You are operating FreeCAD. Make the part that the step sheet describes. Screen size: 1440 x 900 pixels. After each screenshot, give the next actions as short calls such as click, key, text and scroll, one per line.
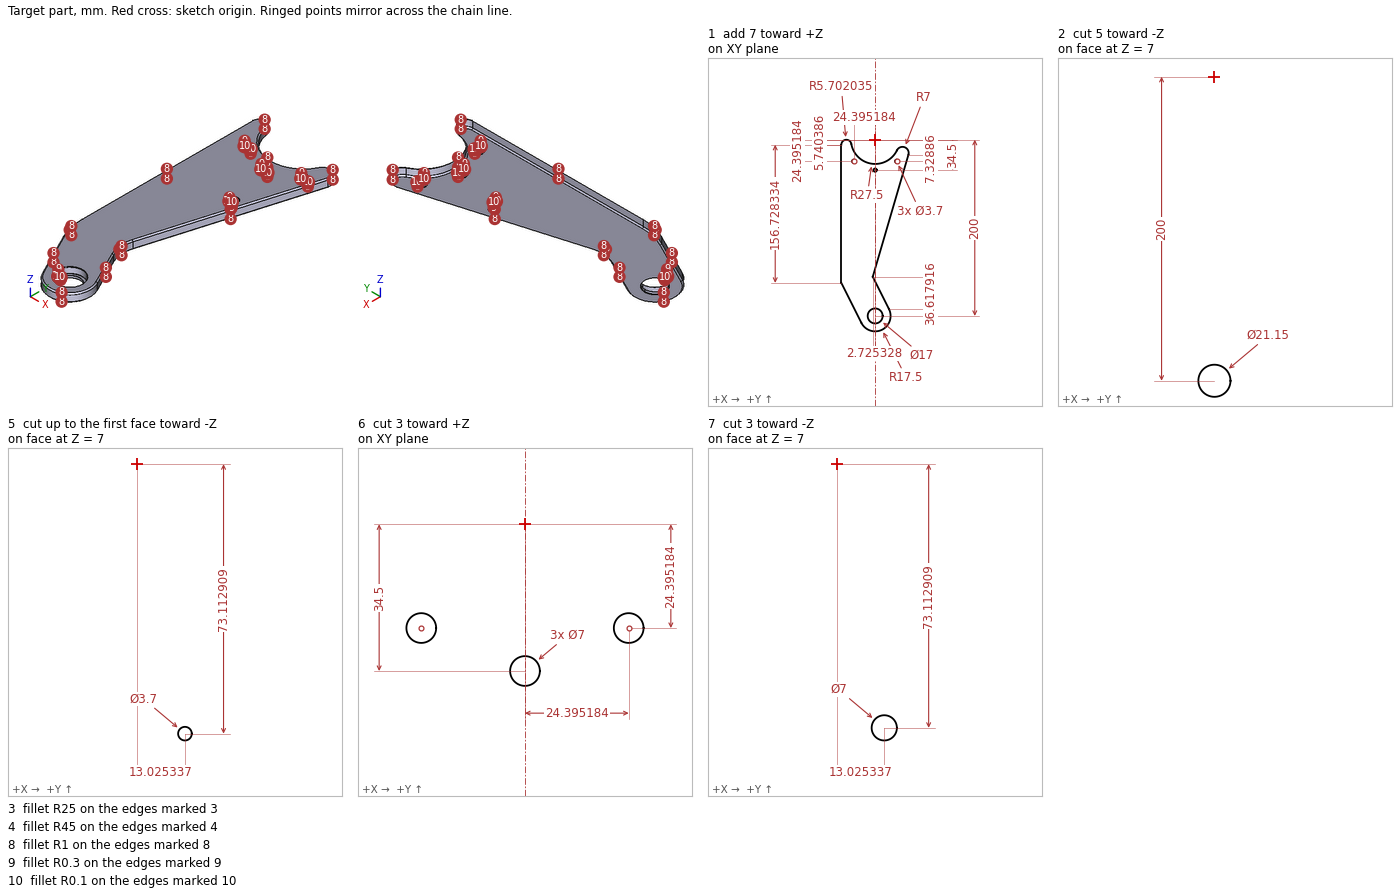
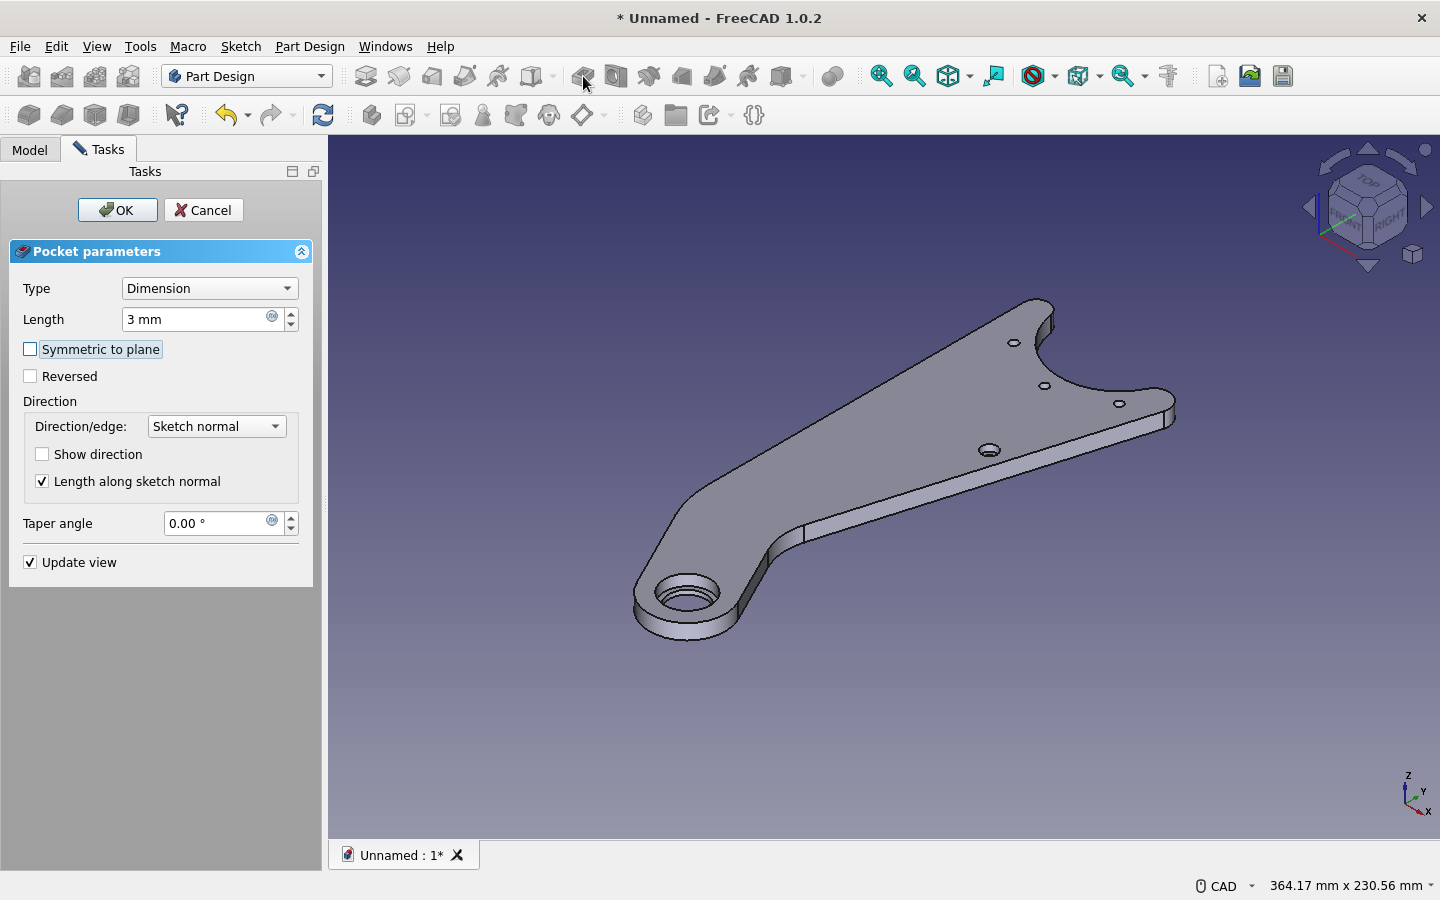
click(118, 210)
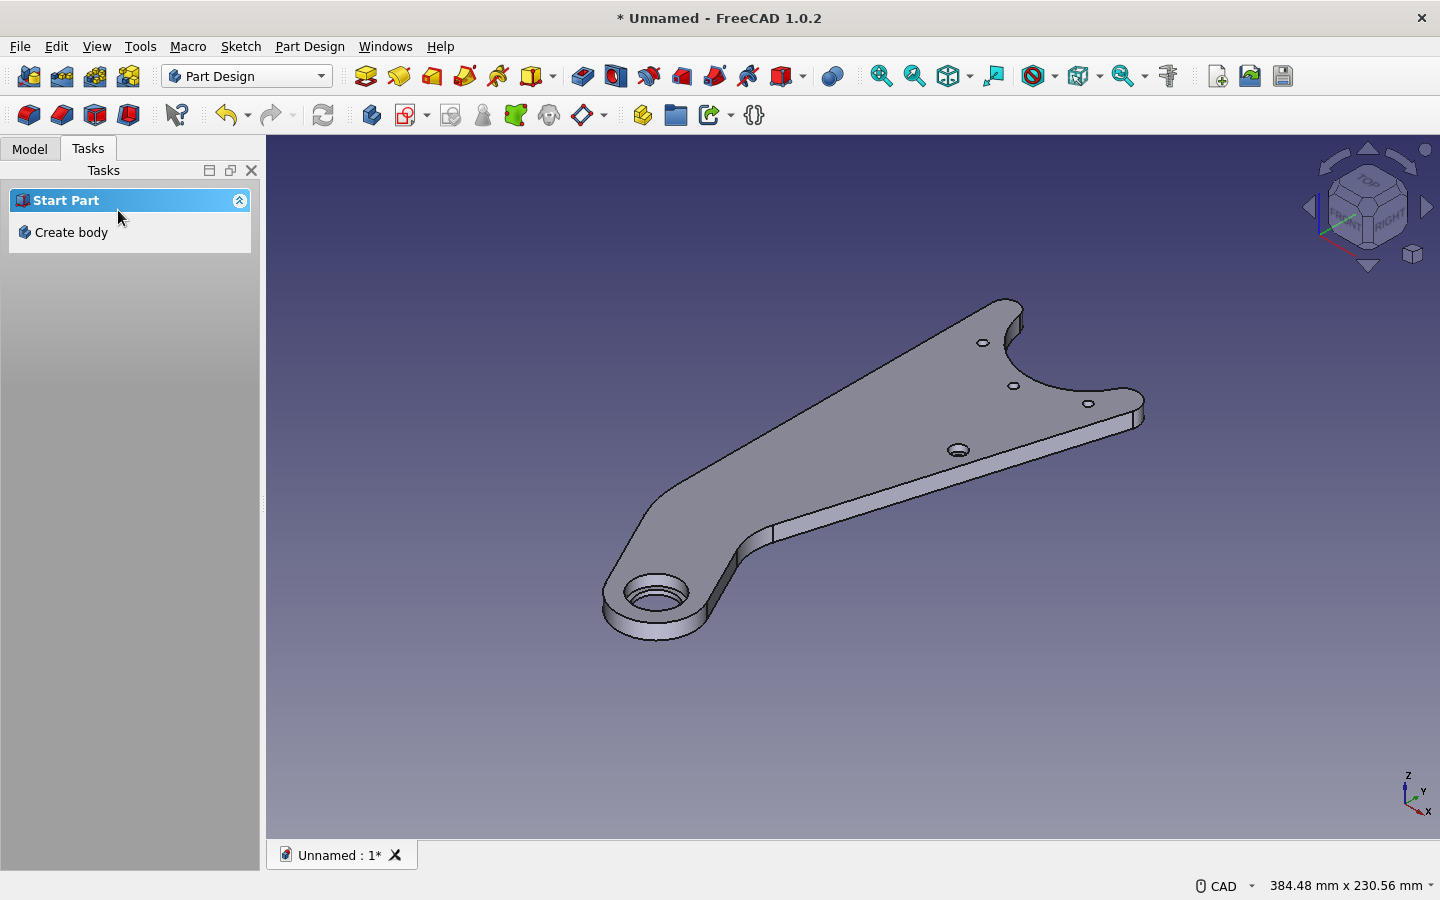
click(613, 627)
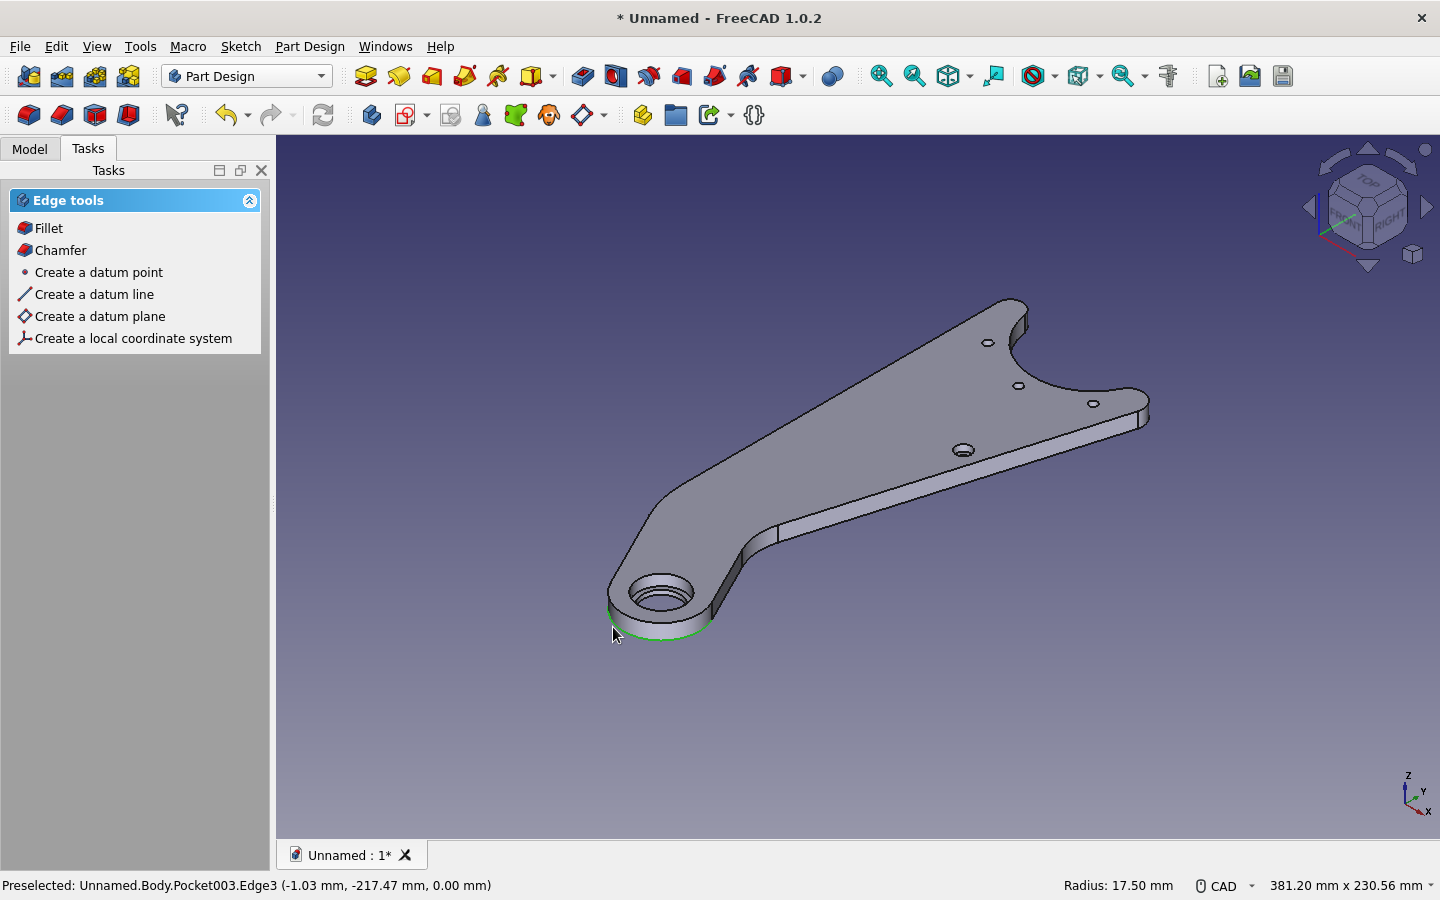
click(958, 467, ctrl)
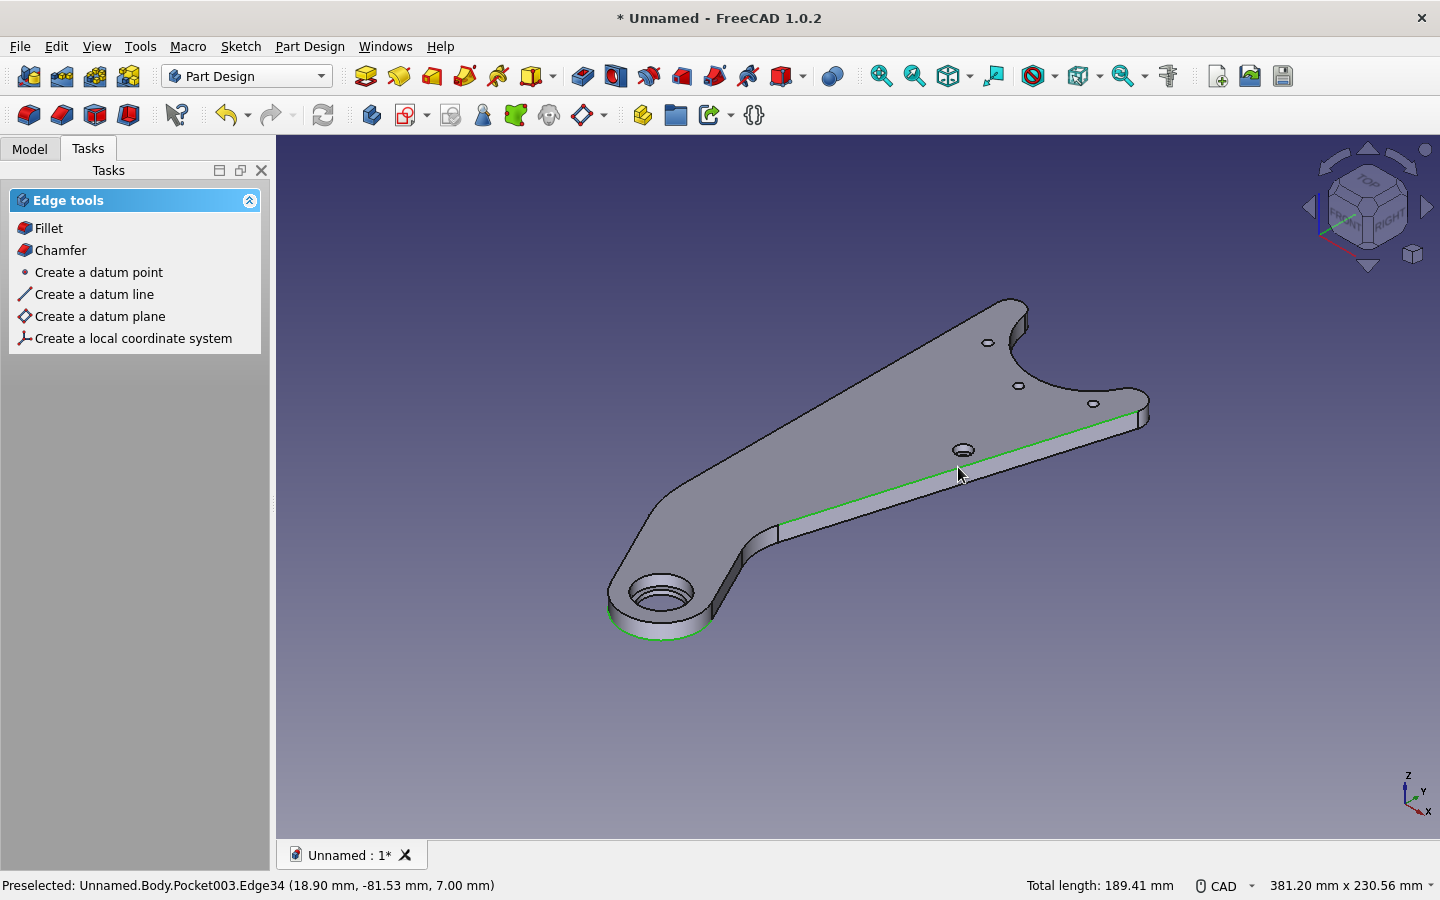
click(1149, 398, ctrl)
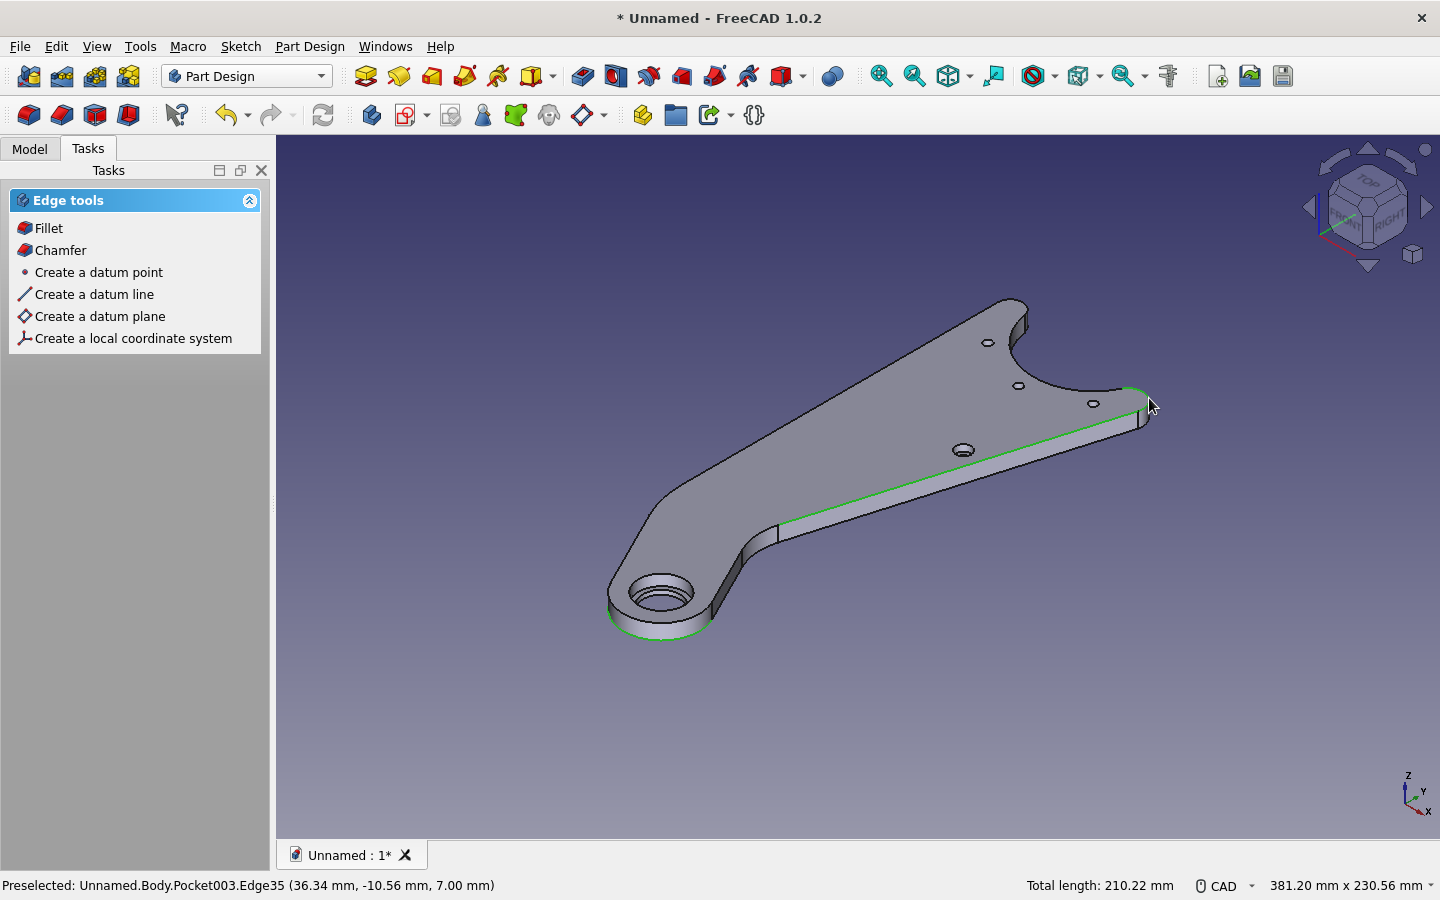
click(1010, 337, ctrl)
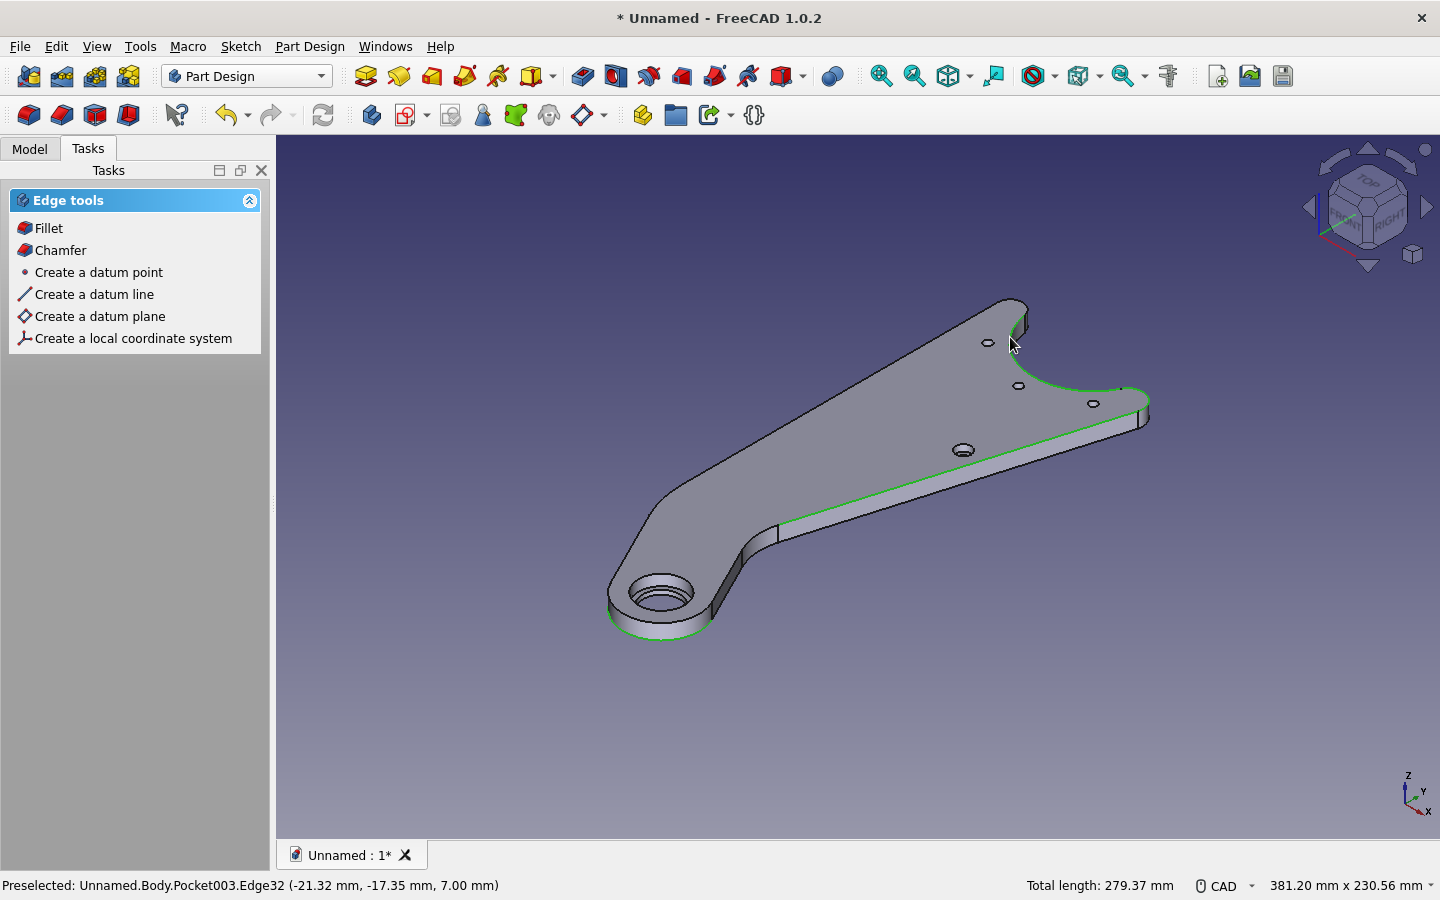
click(1025, 303, ctrl)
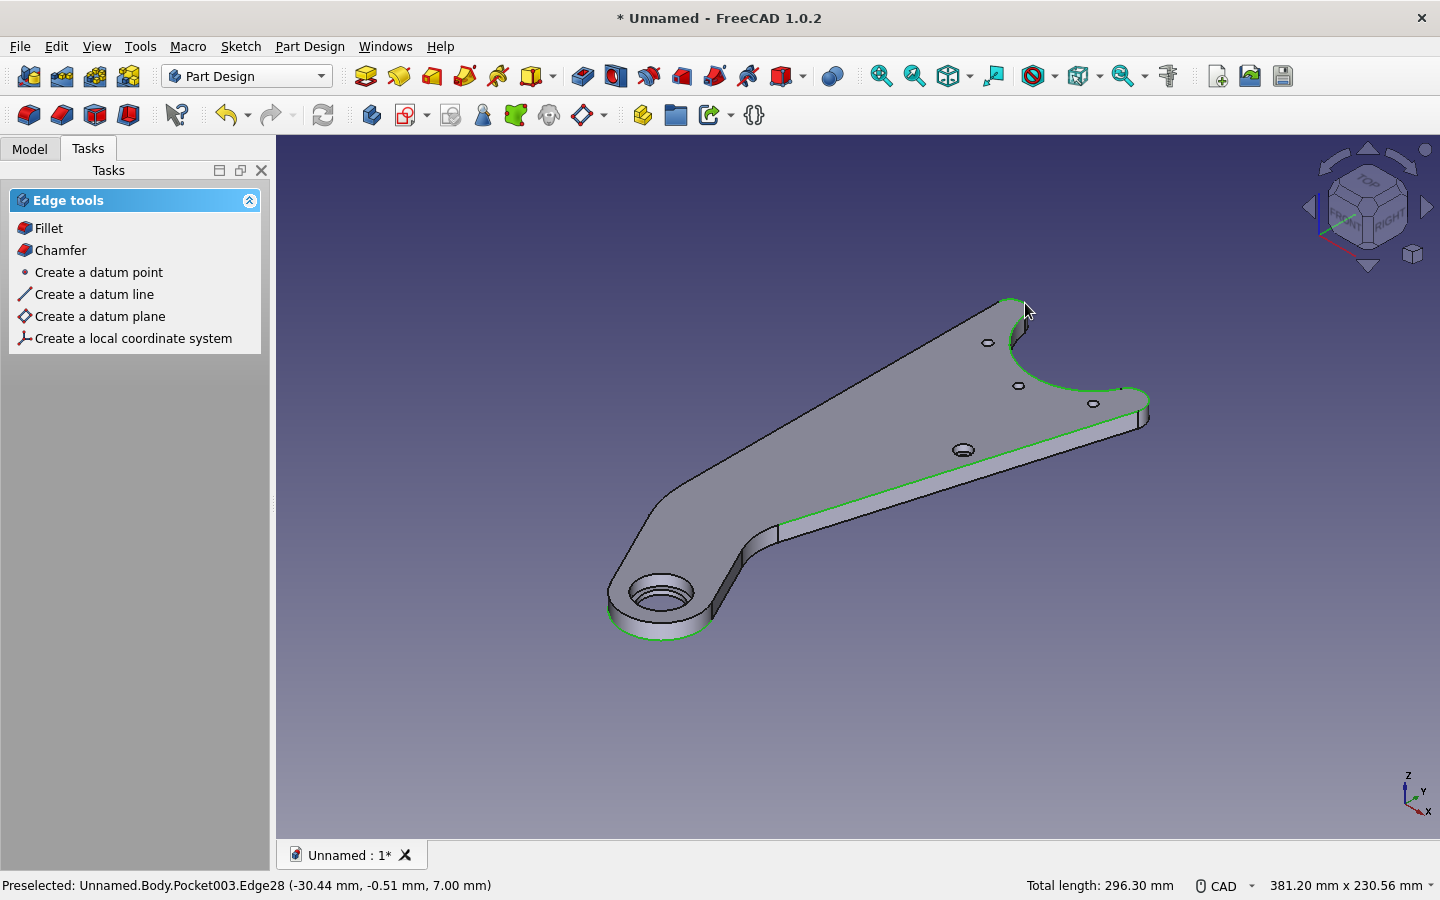
click(727, 575, ctrl)